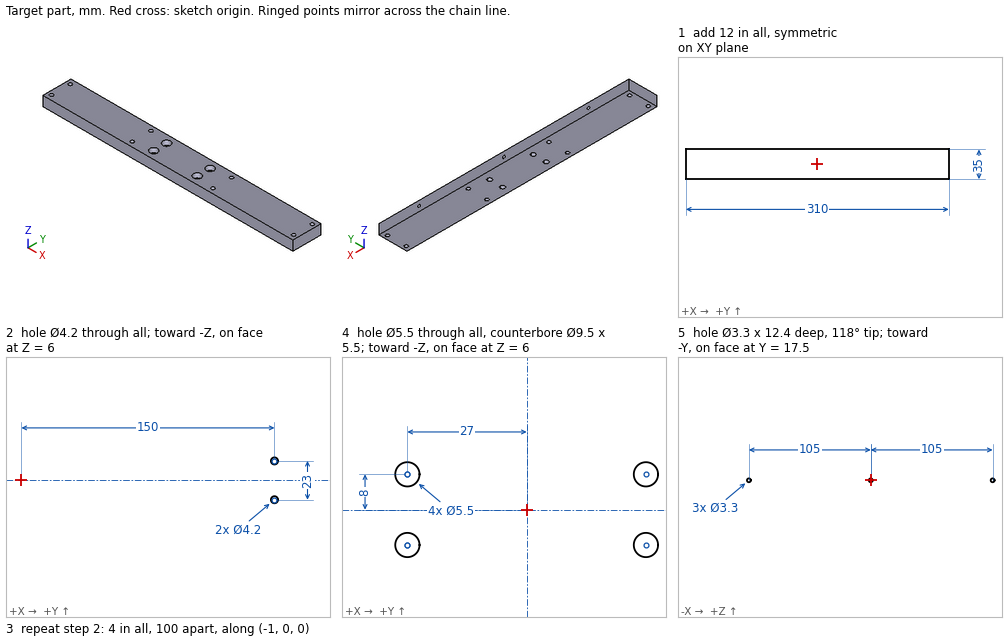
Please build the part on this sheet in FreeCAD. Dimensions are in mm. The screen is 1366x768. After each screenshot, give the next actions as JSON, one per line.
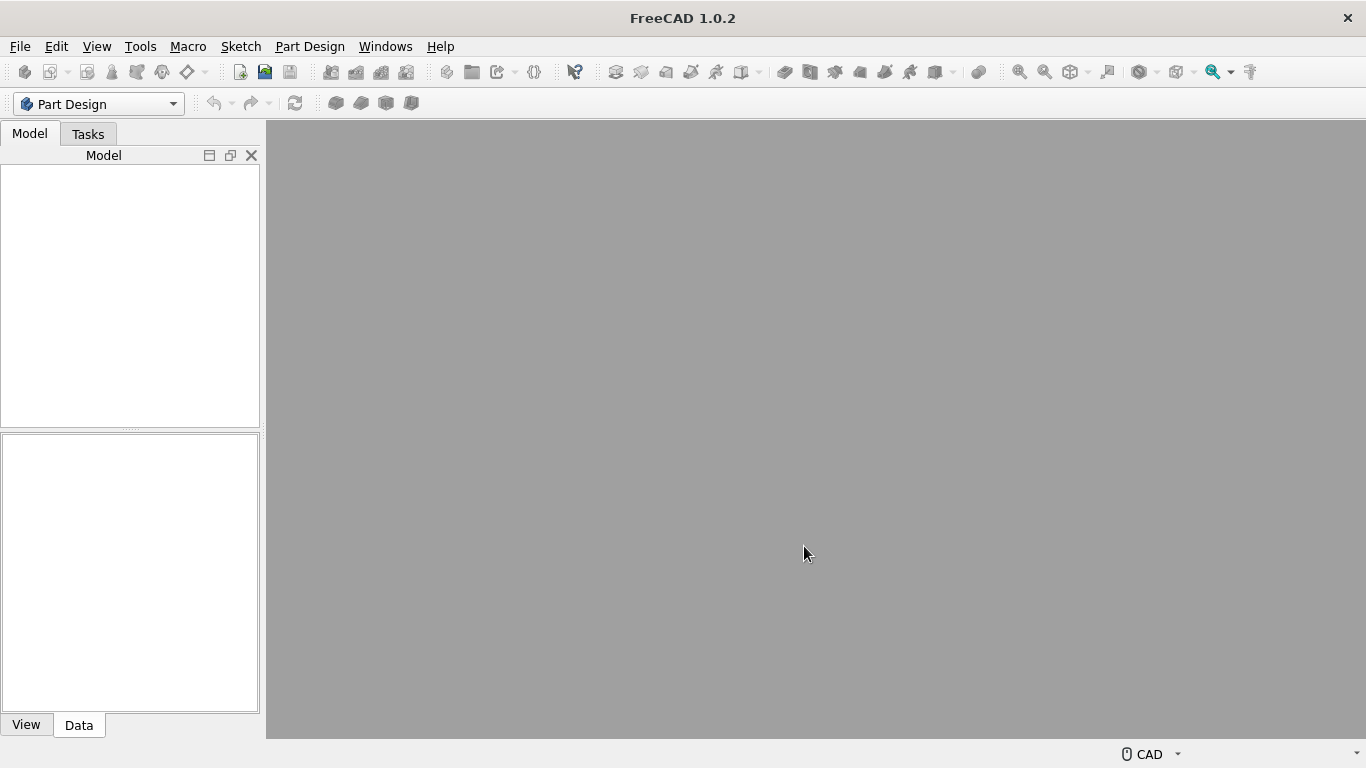
{"action": "left_click", "coordinate": [240, 72]}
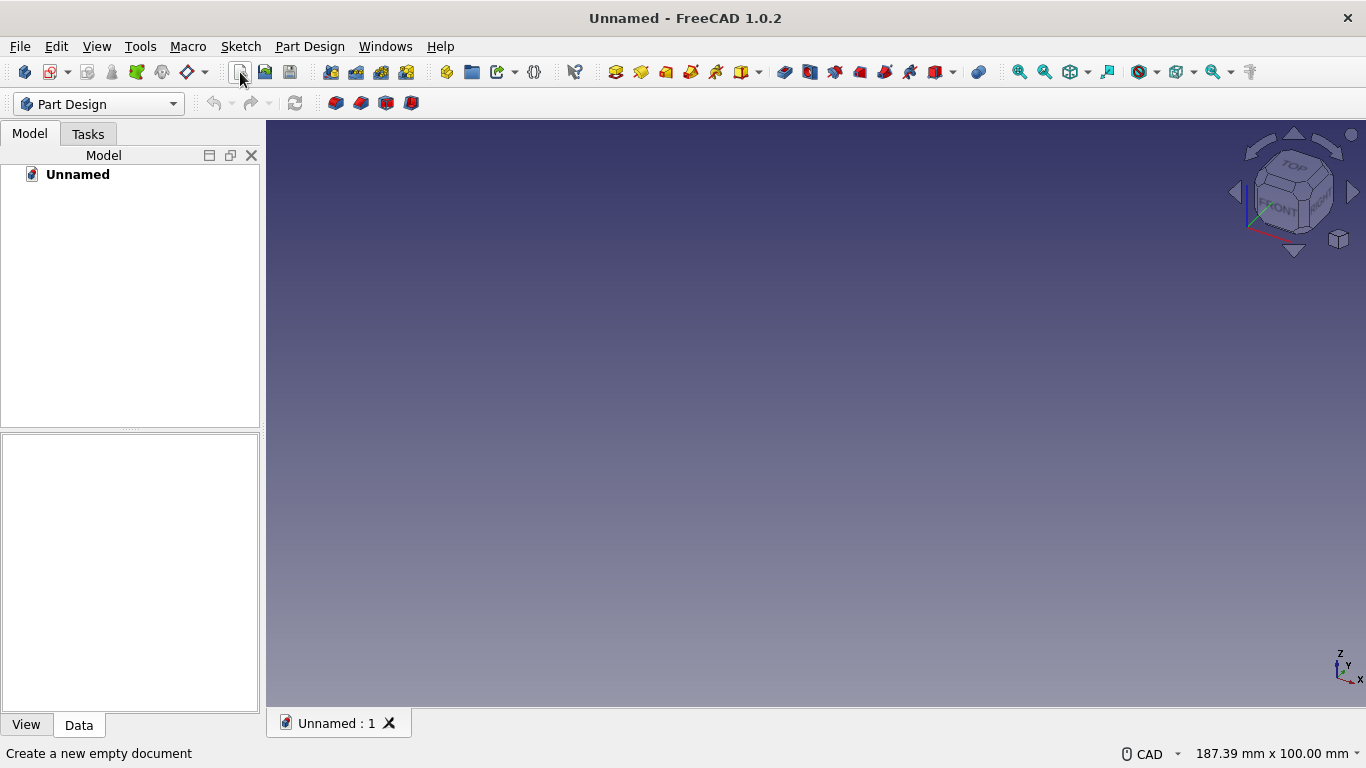
{"action": "left_click", "coordinate": [50, 72]}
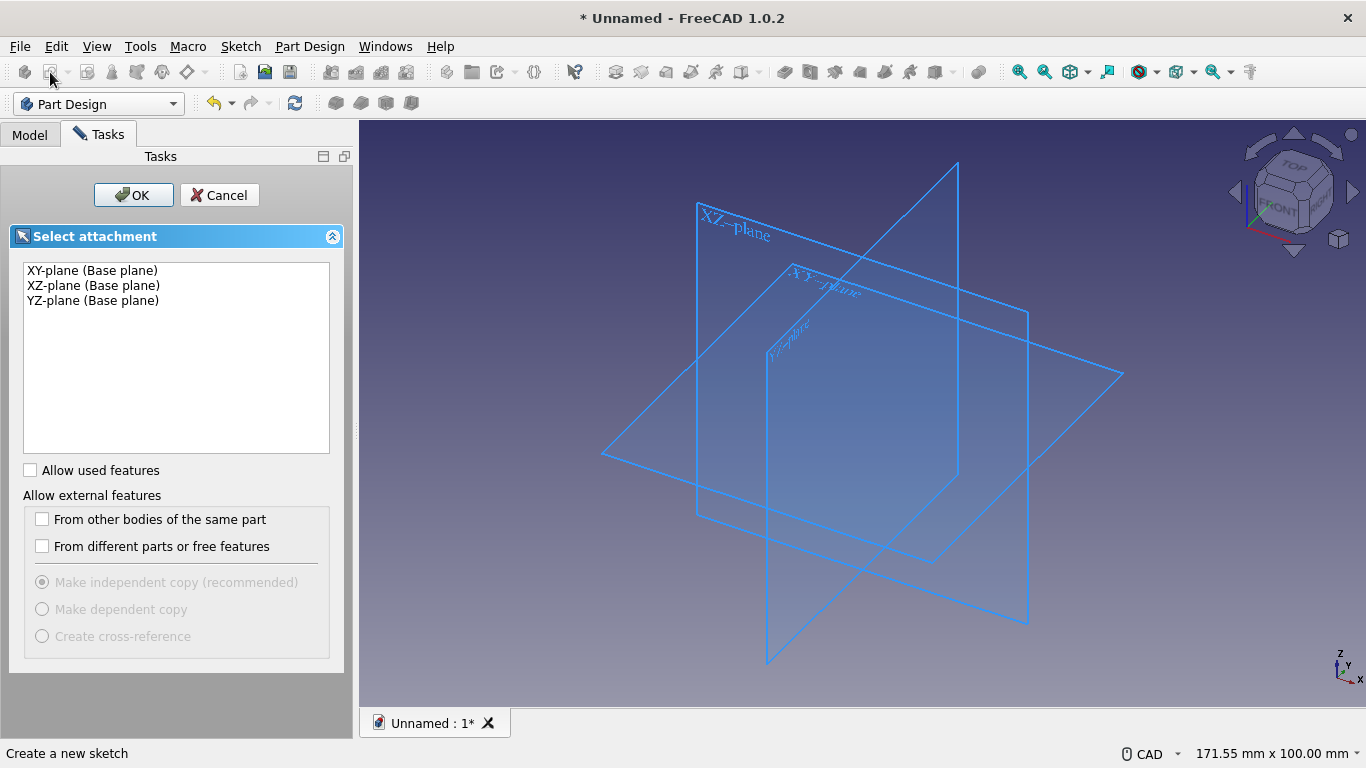
{"action": "left_click", "coordinate": [84, 270]}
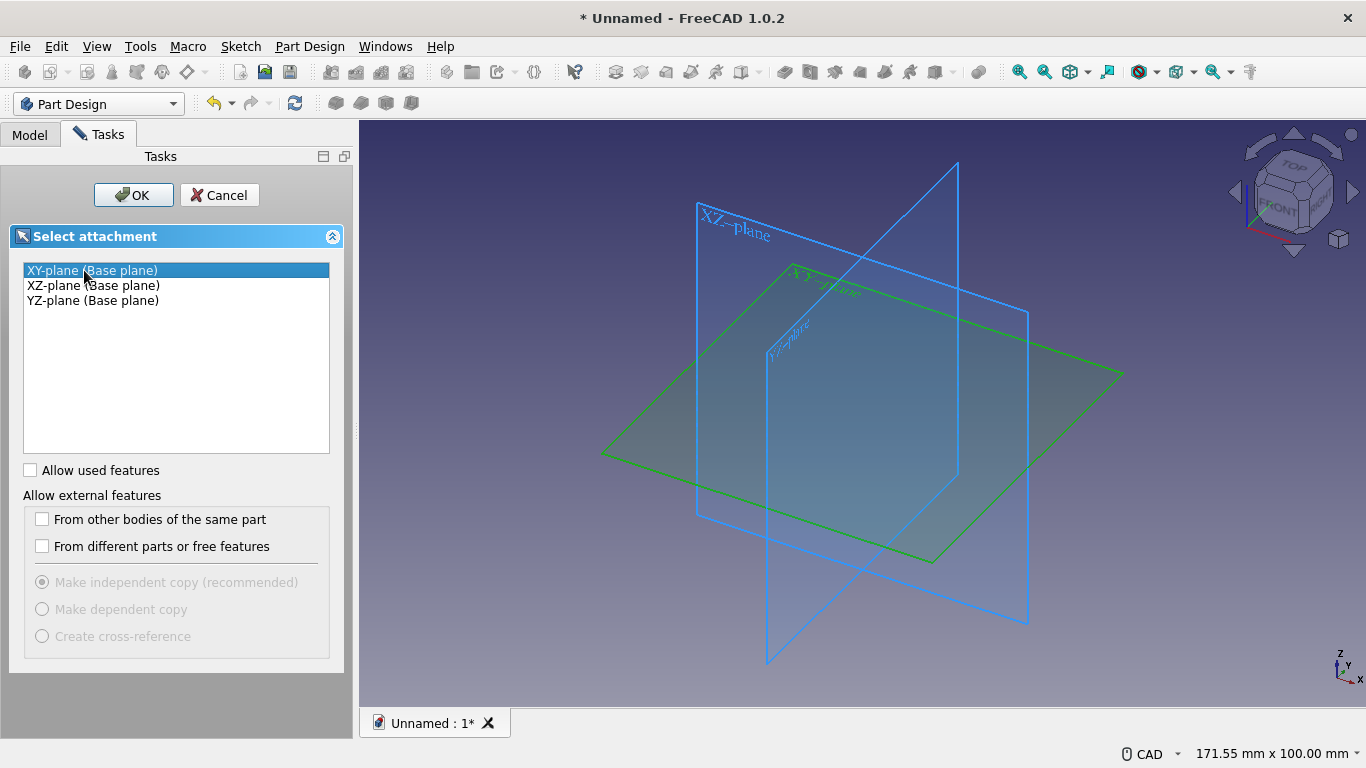
{"action": "left_click", "coordinate": [134, 195]}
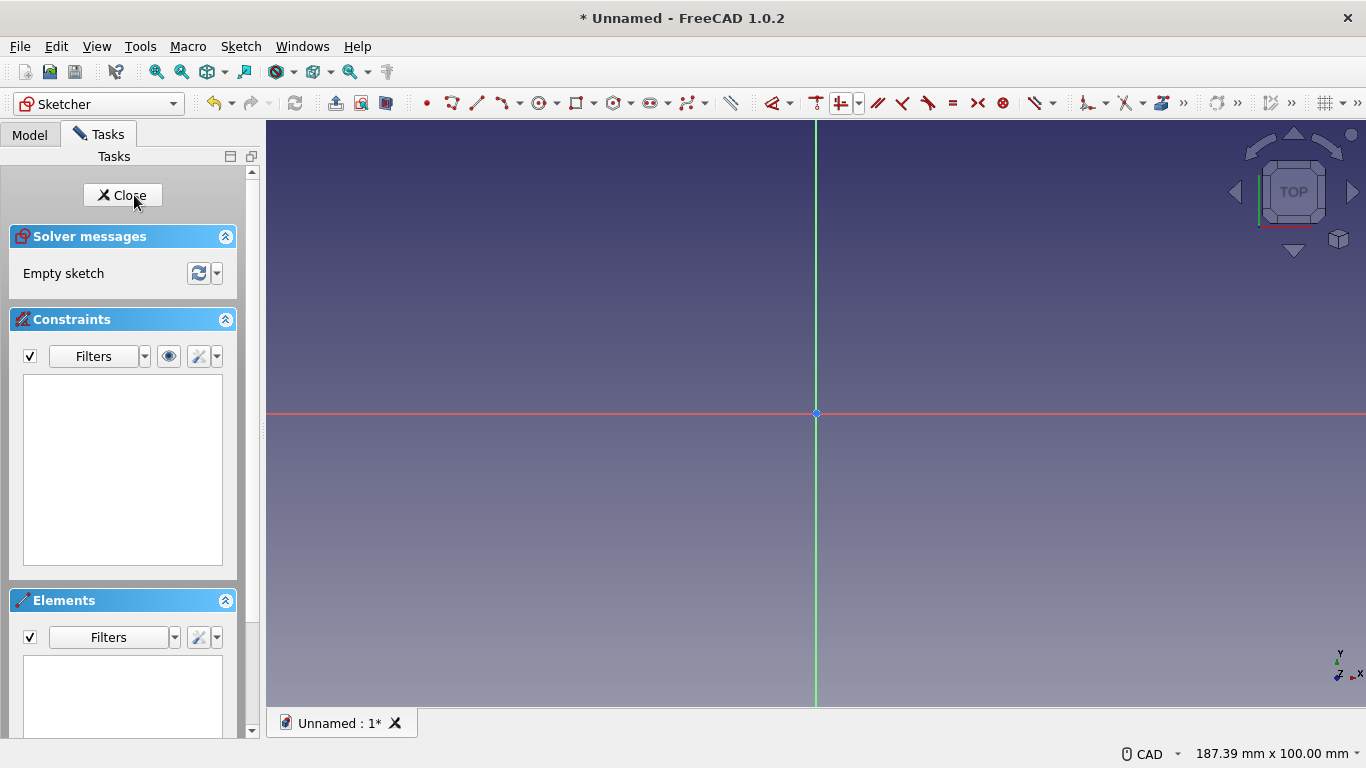
{"action": "scroll", "coordinate": [708, 414], "scroll_direction": "down", "scroll_amount": 5}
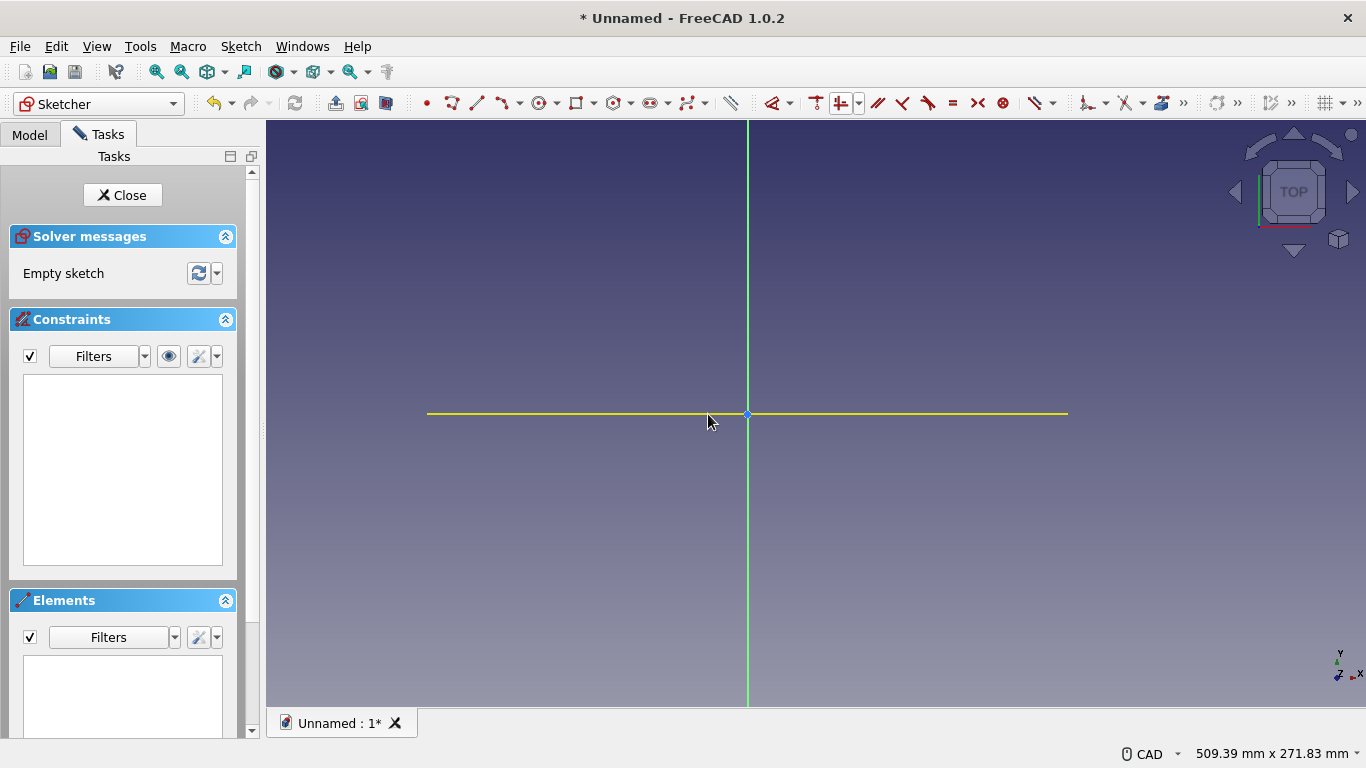
{"action": "left_click", "coordinate": [594, 104]}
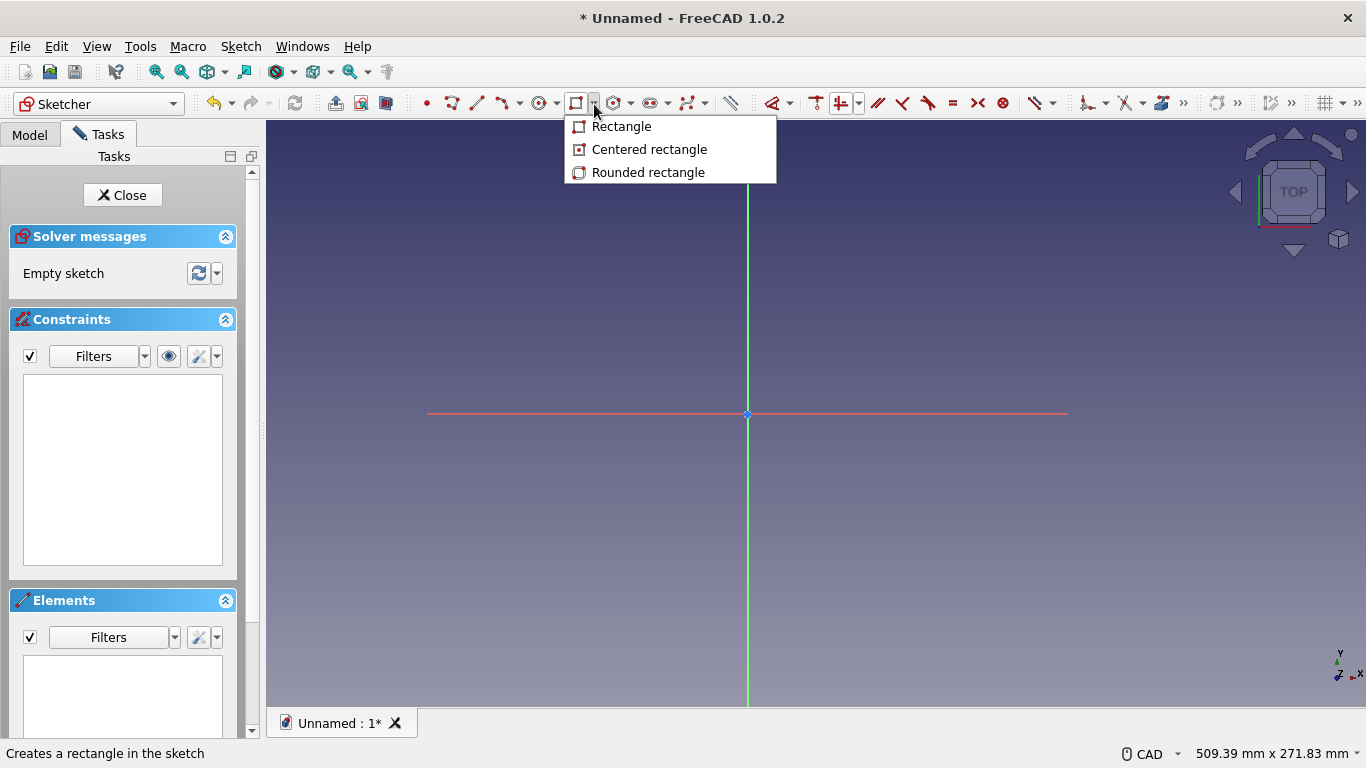
{"action": "left_click", "coordinate": [670, 150]}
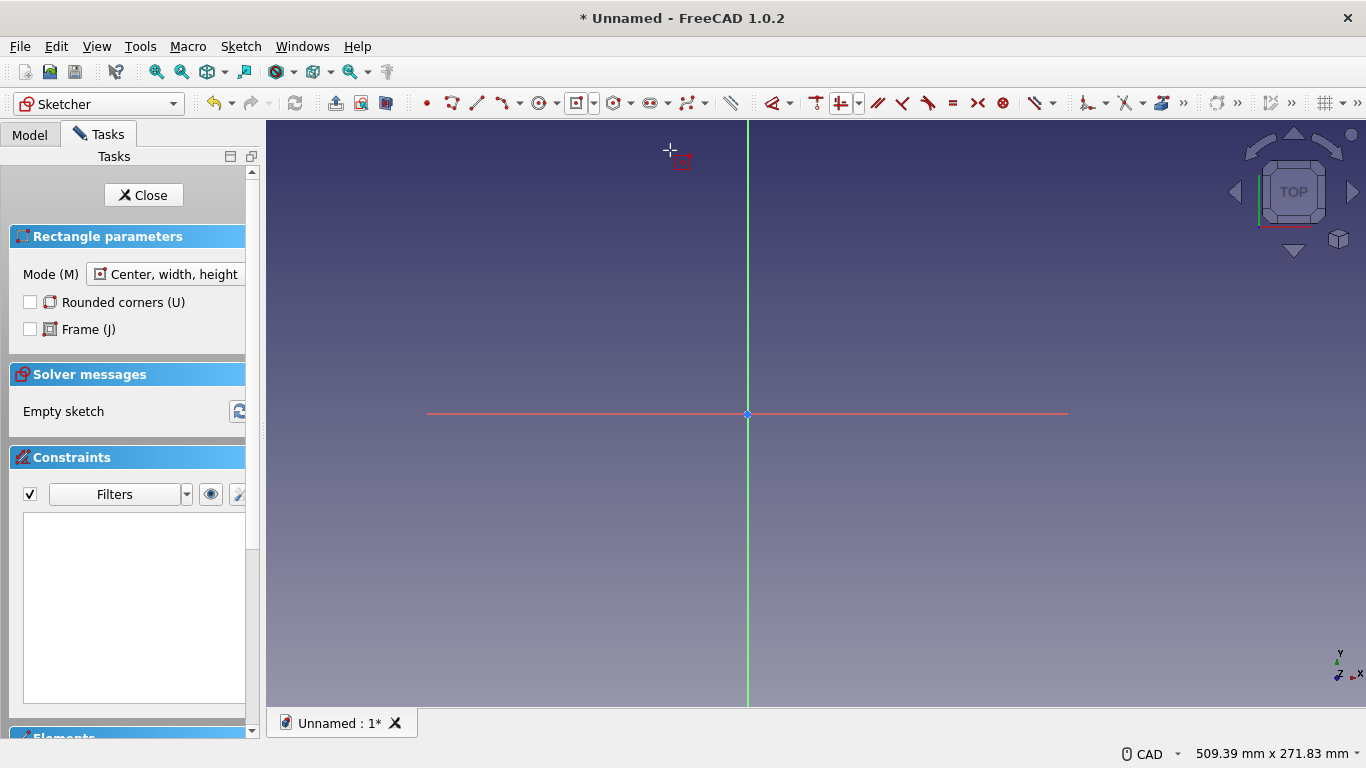
{"action": "left_click", "coordinate": [748, 414]}
{"action": "left_click", "coordinate": [1083, 376]}
{"action": "key", "text": "Escape"}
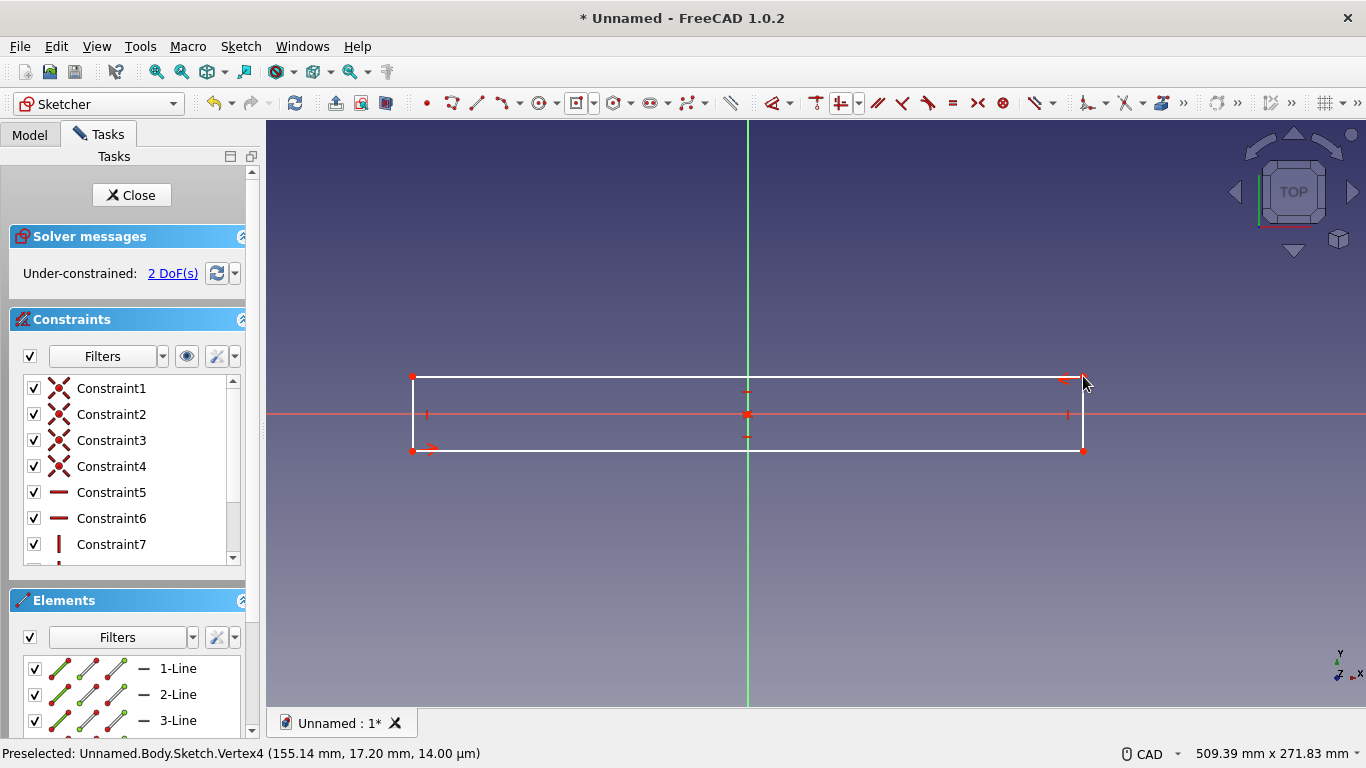
{"action": "left_click", "coordinate": [772, 104]}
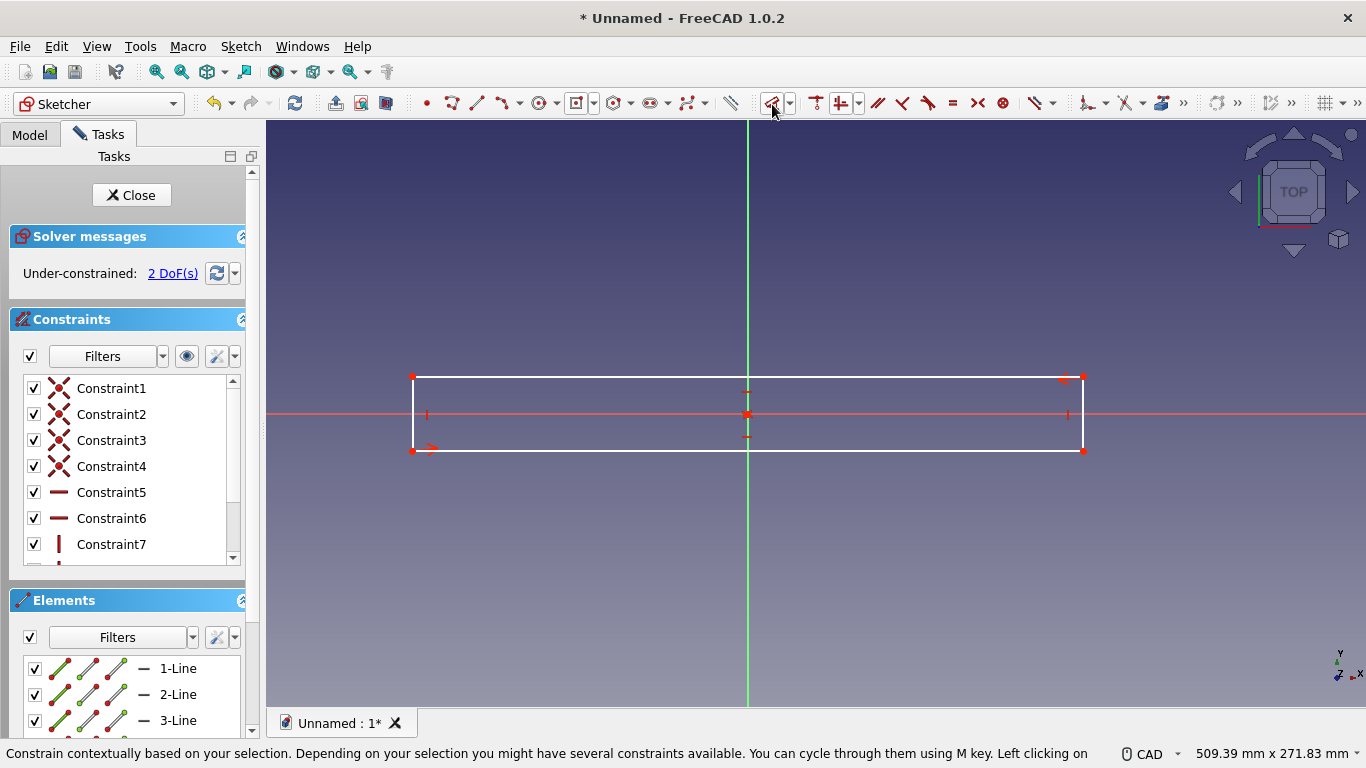
{"action": "left_click", "coordinate": [1083, 429]}
{"action": "left_click", "coordinate": [1117, 397]}